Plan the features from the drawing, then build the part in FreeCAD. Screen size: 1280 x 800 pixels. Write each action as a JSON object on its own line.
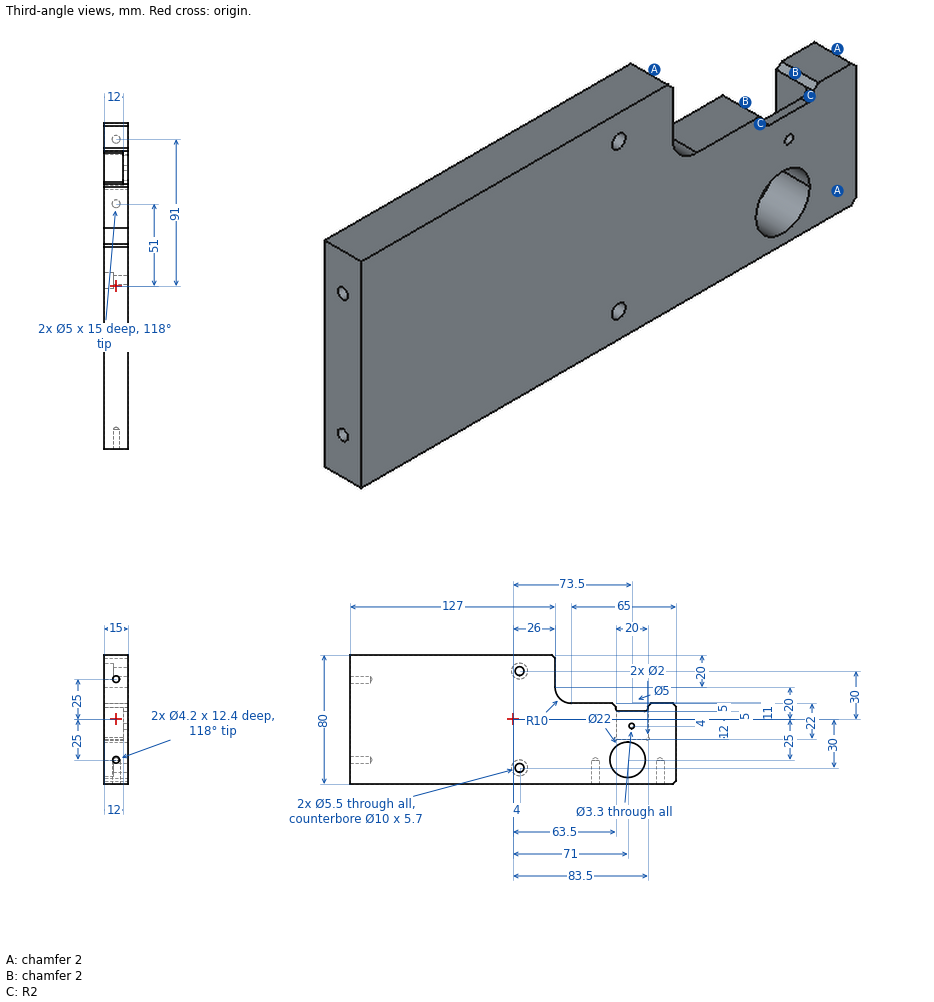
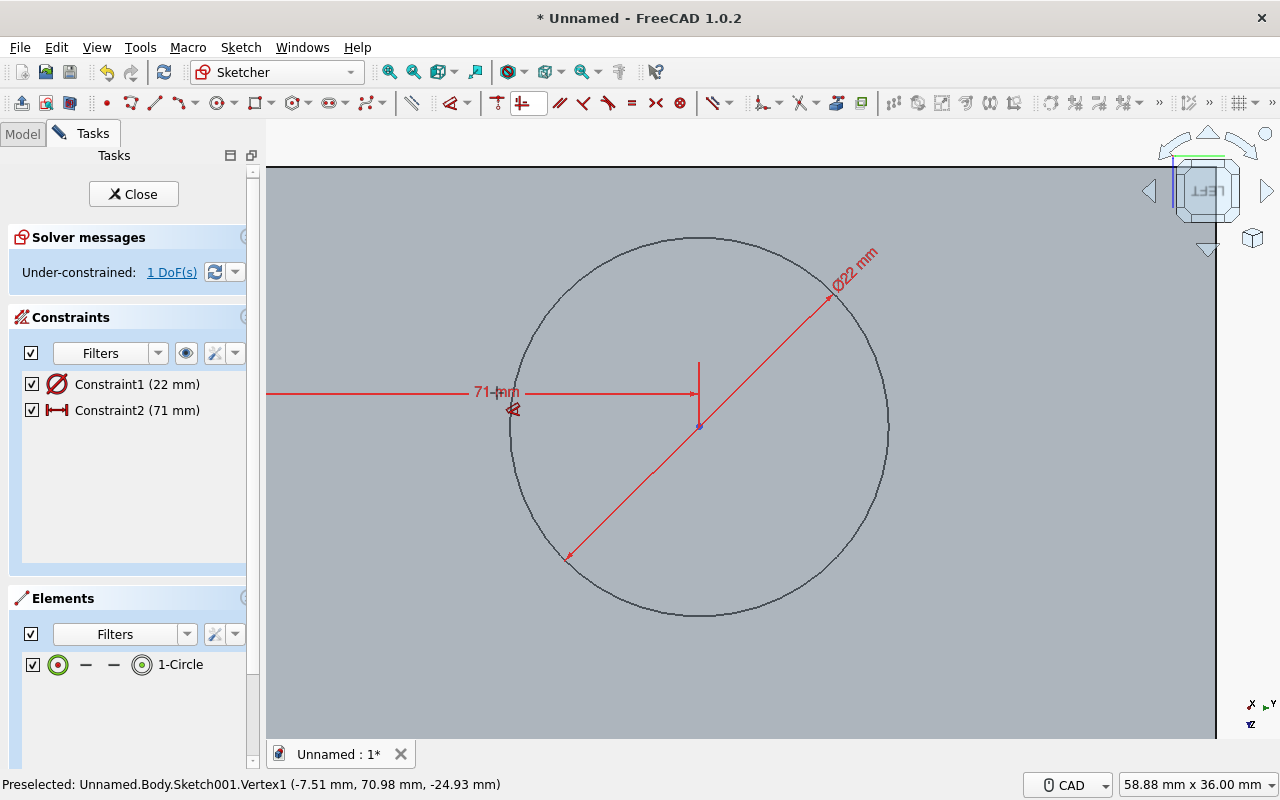
{"action": "left_click", "coordinate": [699, 427]}
{"action": "left_click", "coordinate": [733, 569]}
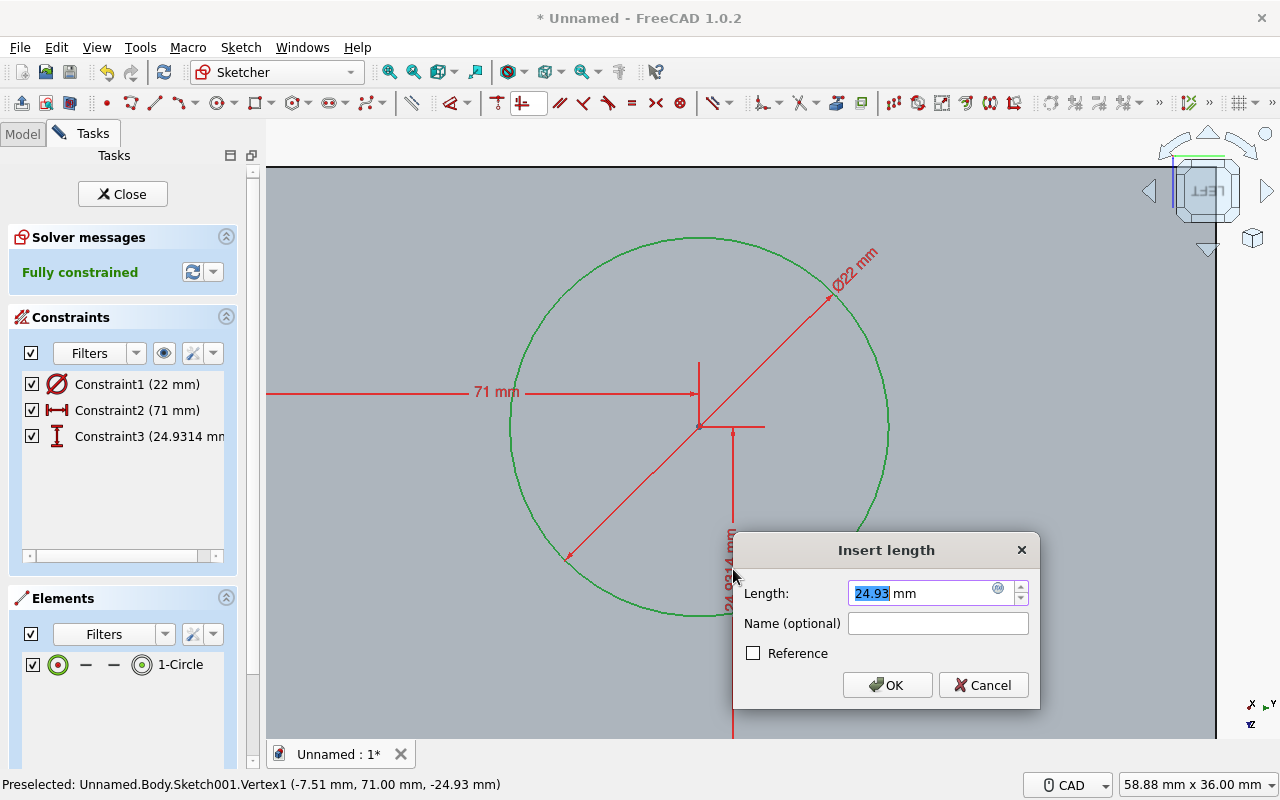
{"action": "type", "text": "25"}
{"action": "key", "text": "Return"}
{"action": "key", "text": "Escape"}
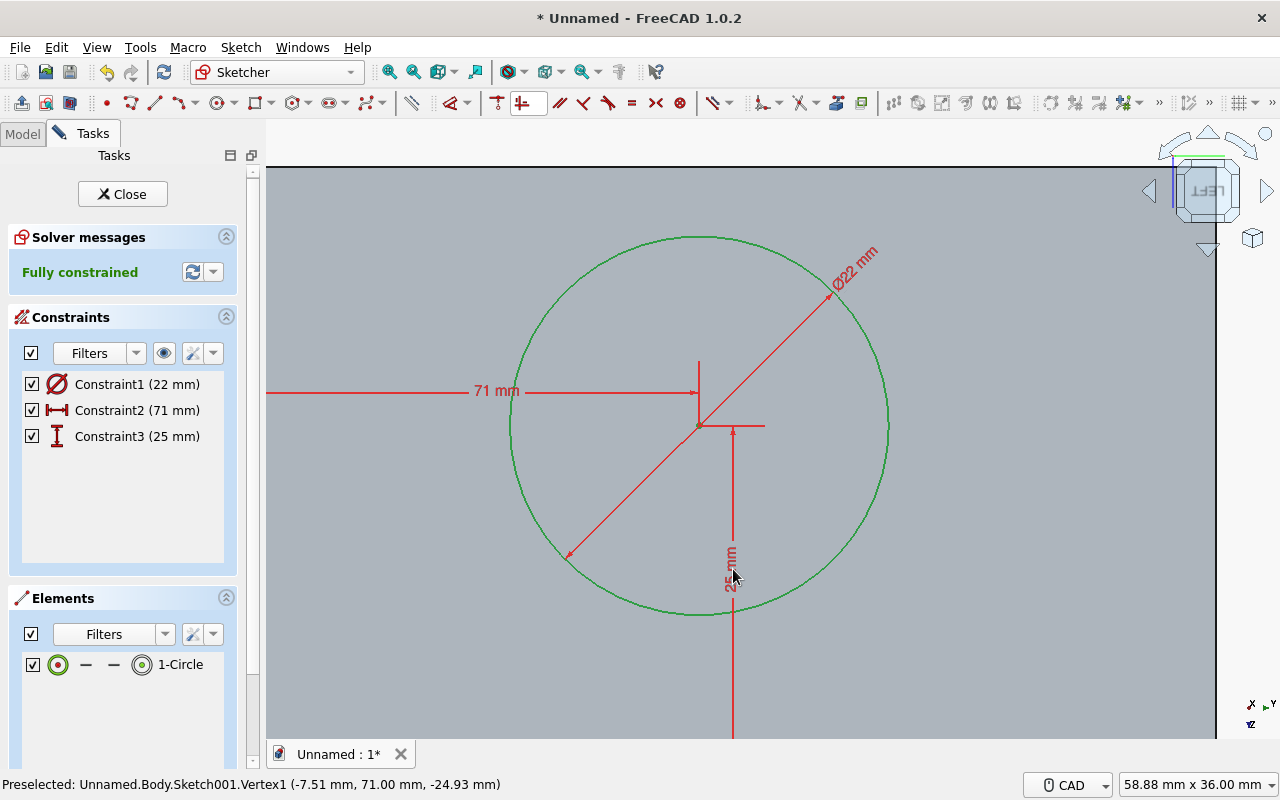
{"action": "left_click", "coordinate": [123, 194]}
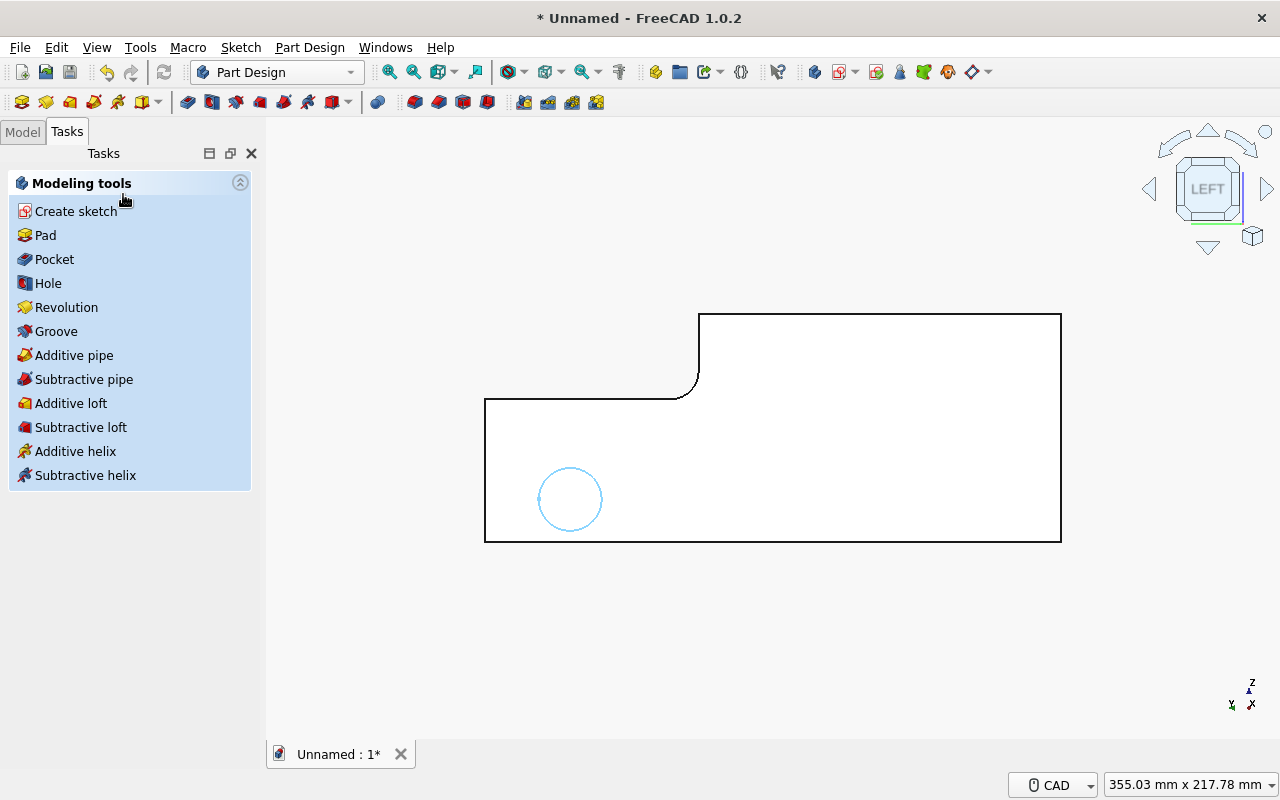
{"action": "left_click", "coordinate": [188, 102]}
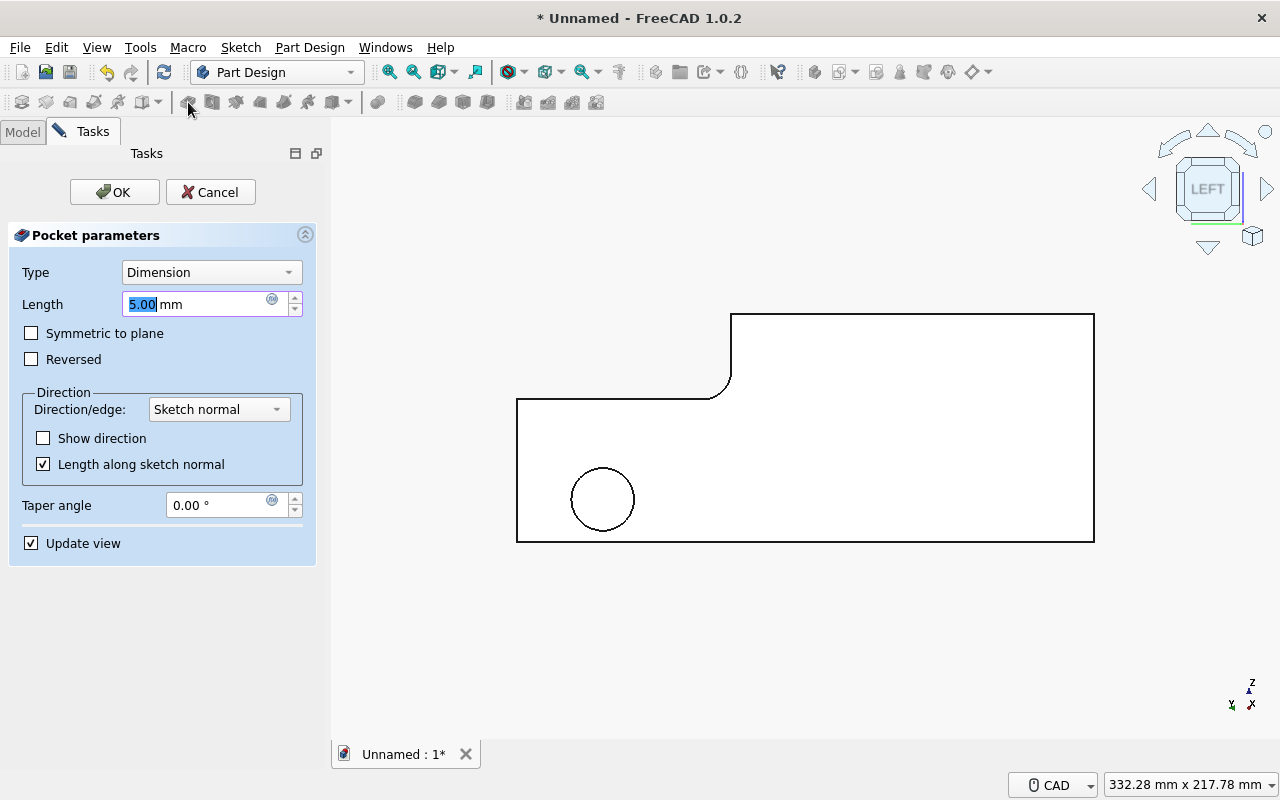
{"action": "left_click", "coordinate": [212, 272]}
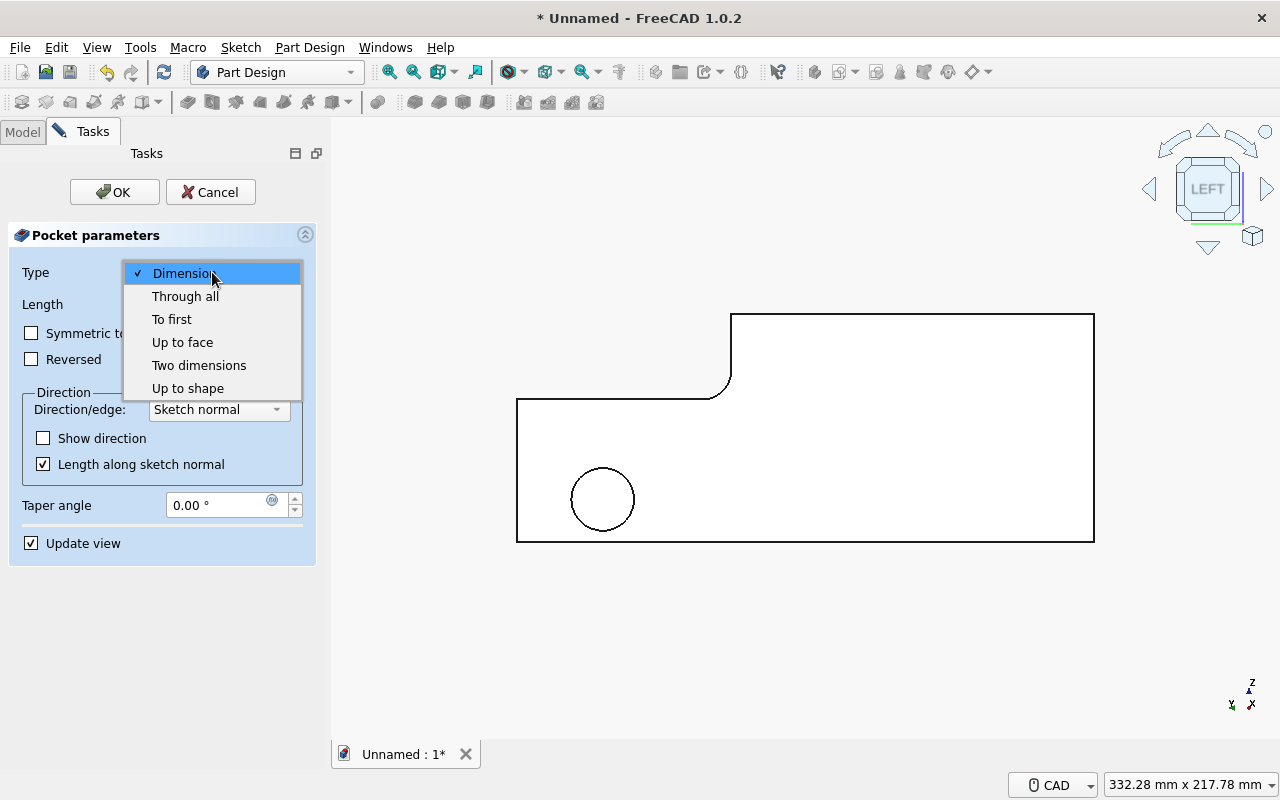
{"action": "left_click", "coordinate": [212, 296]}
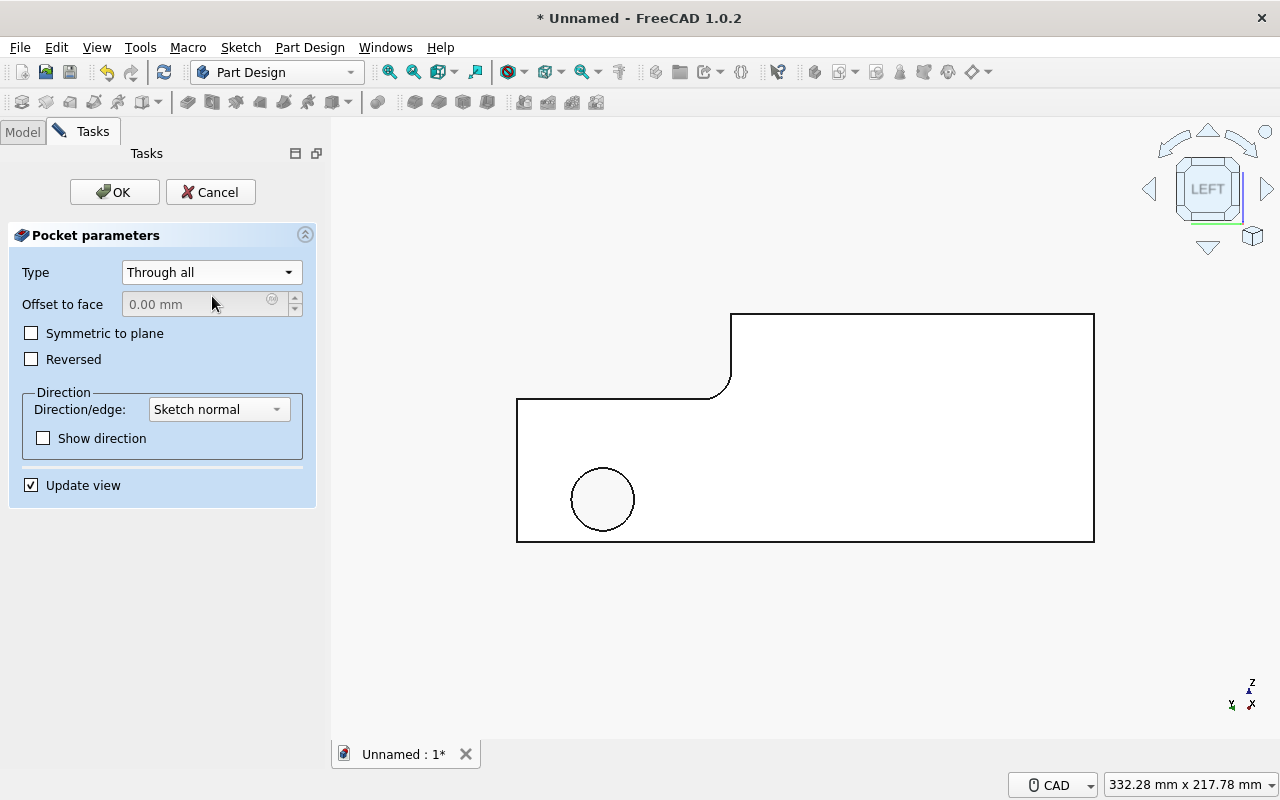
{"action": "left_click", "coordinate": [115, 192]}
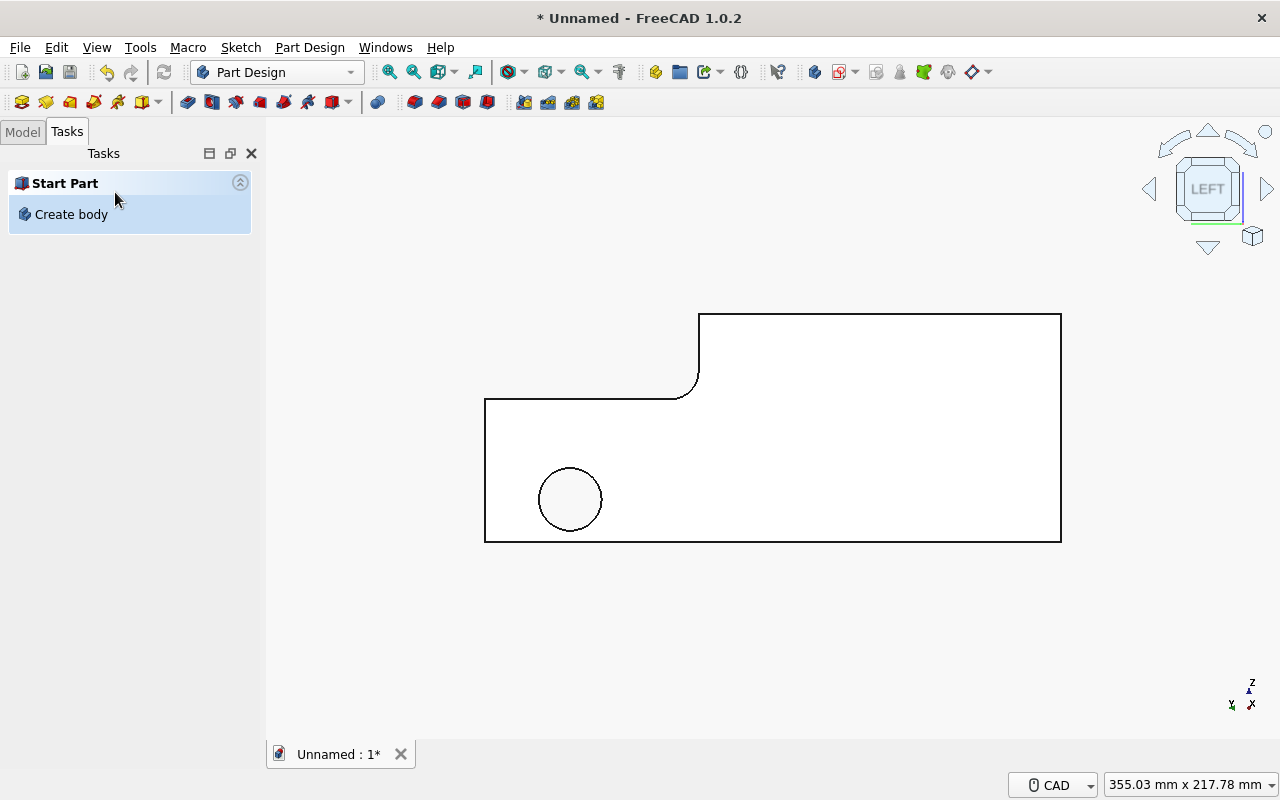
{"action": "key", "text": "0"}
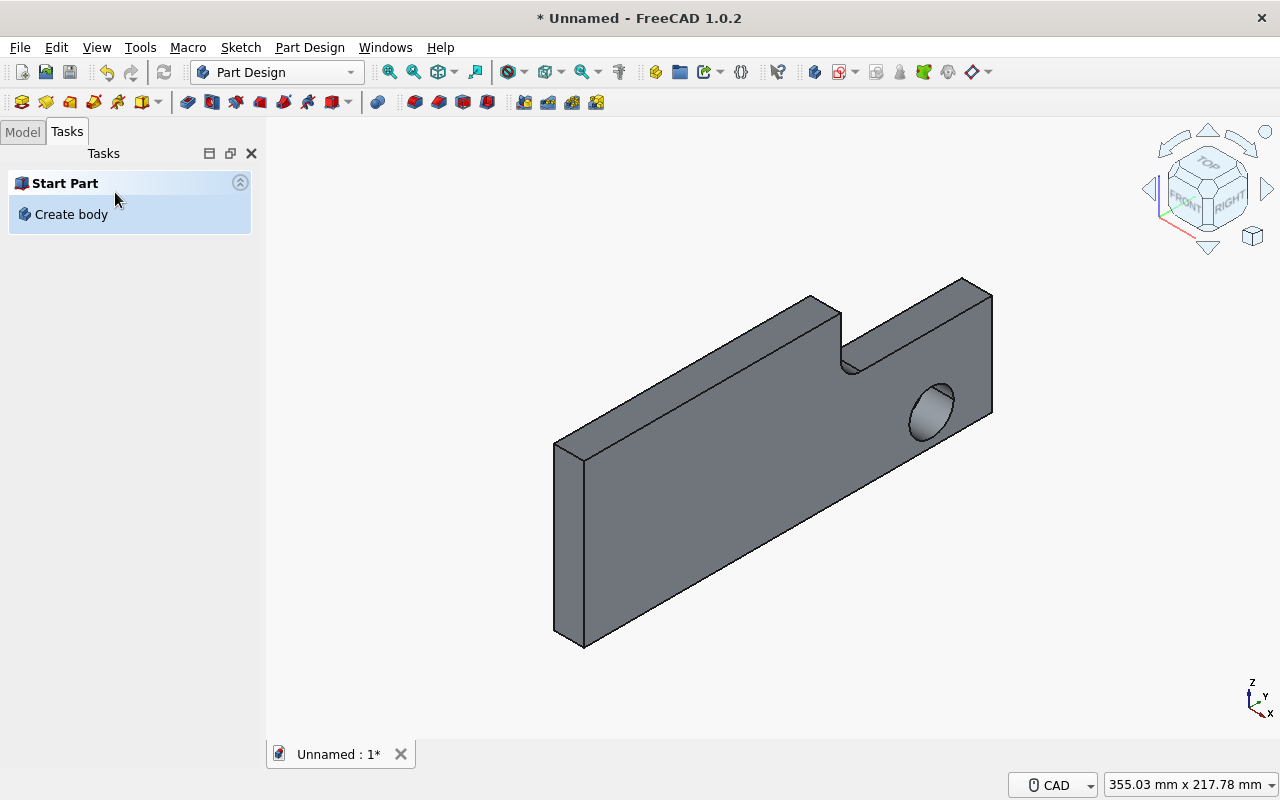
{"action": "left_click", "coordinate": [569, 598]}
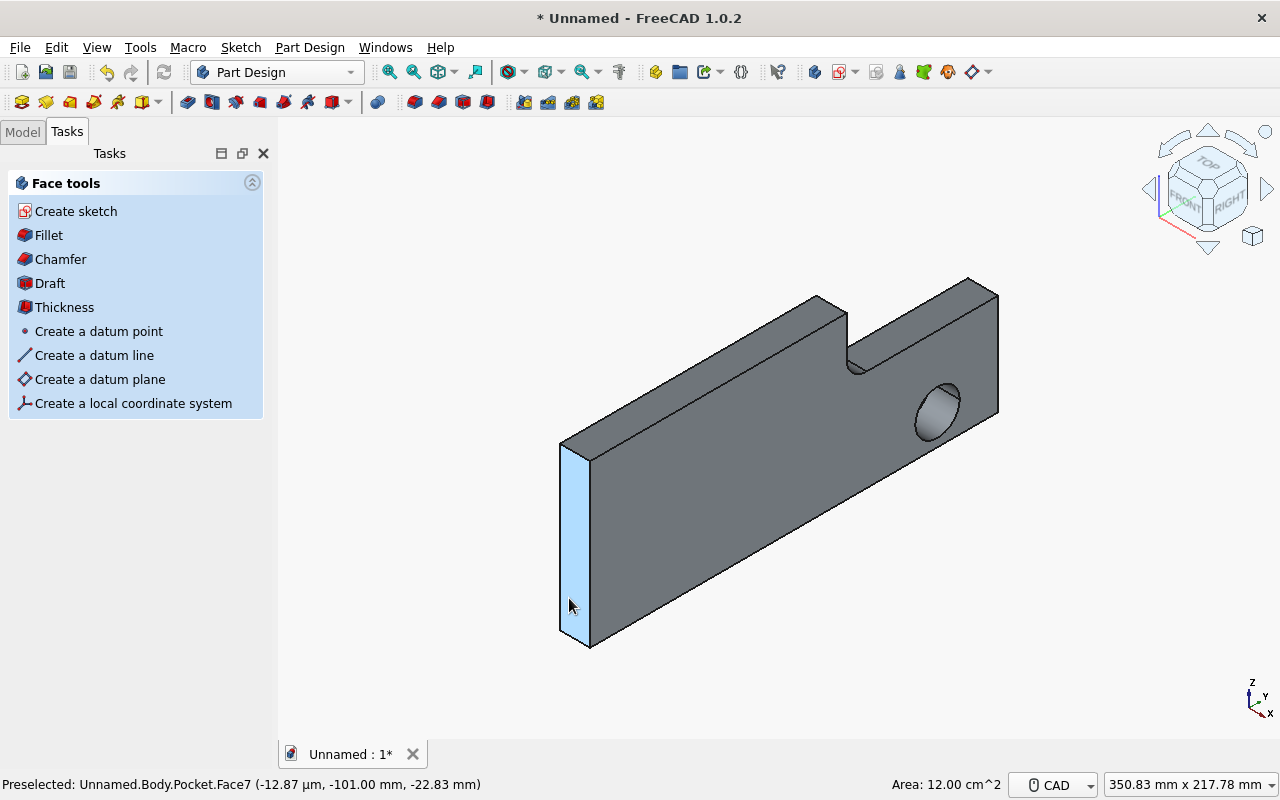
{"action": "left_click", "coordinate": [840, 72]}